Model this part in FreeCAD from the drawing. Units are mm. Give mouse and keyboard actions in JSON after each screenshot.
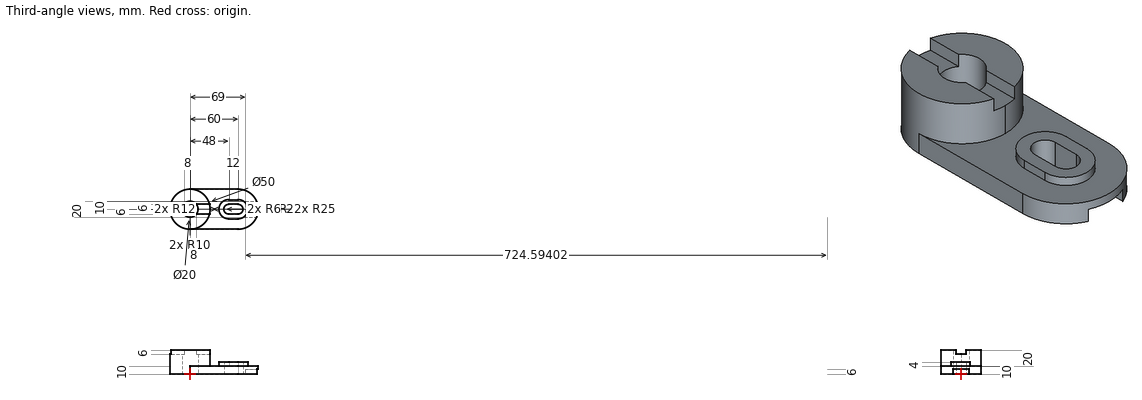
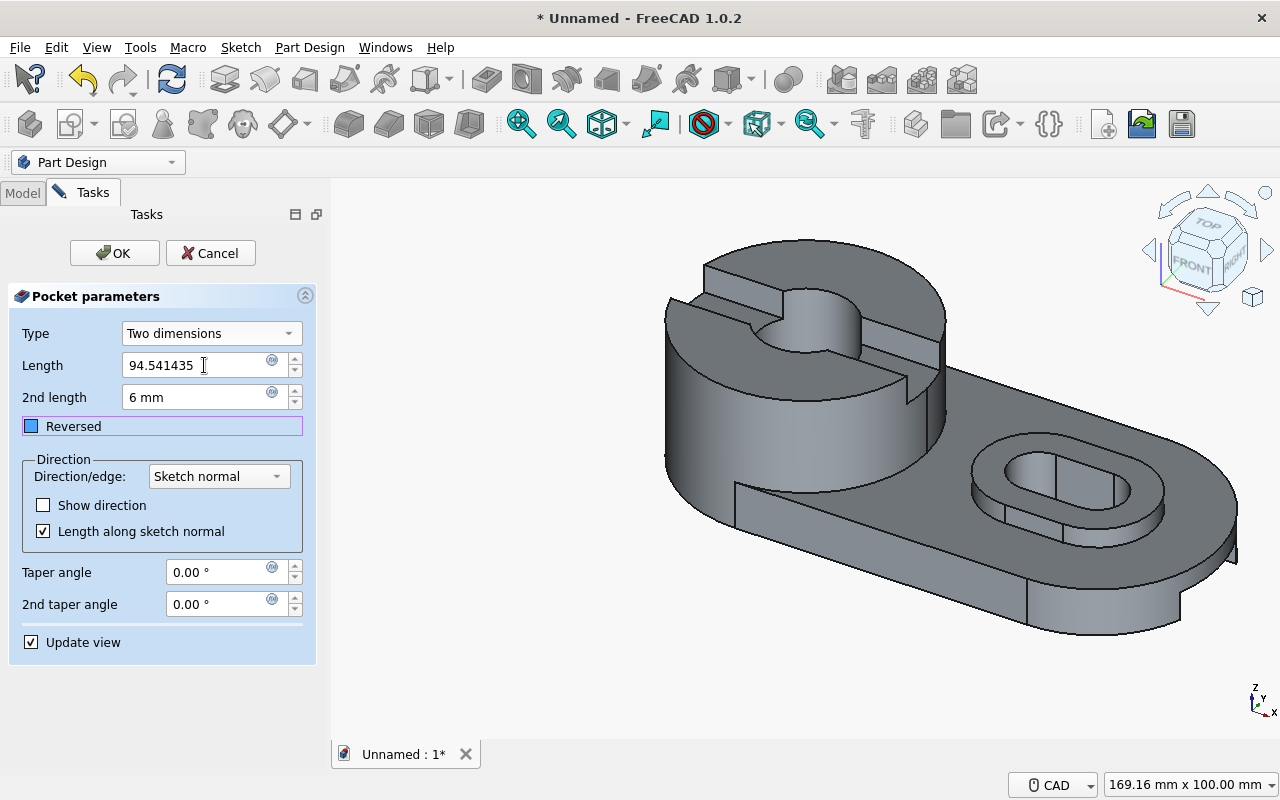
{"action": "left_click", "coordinate": [115, 253]}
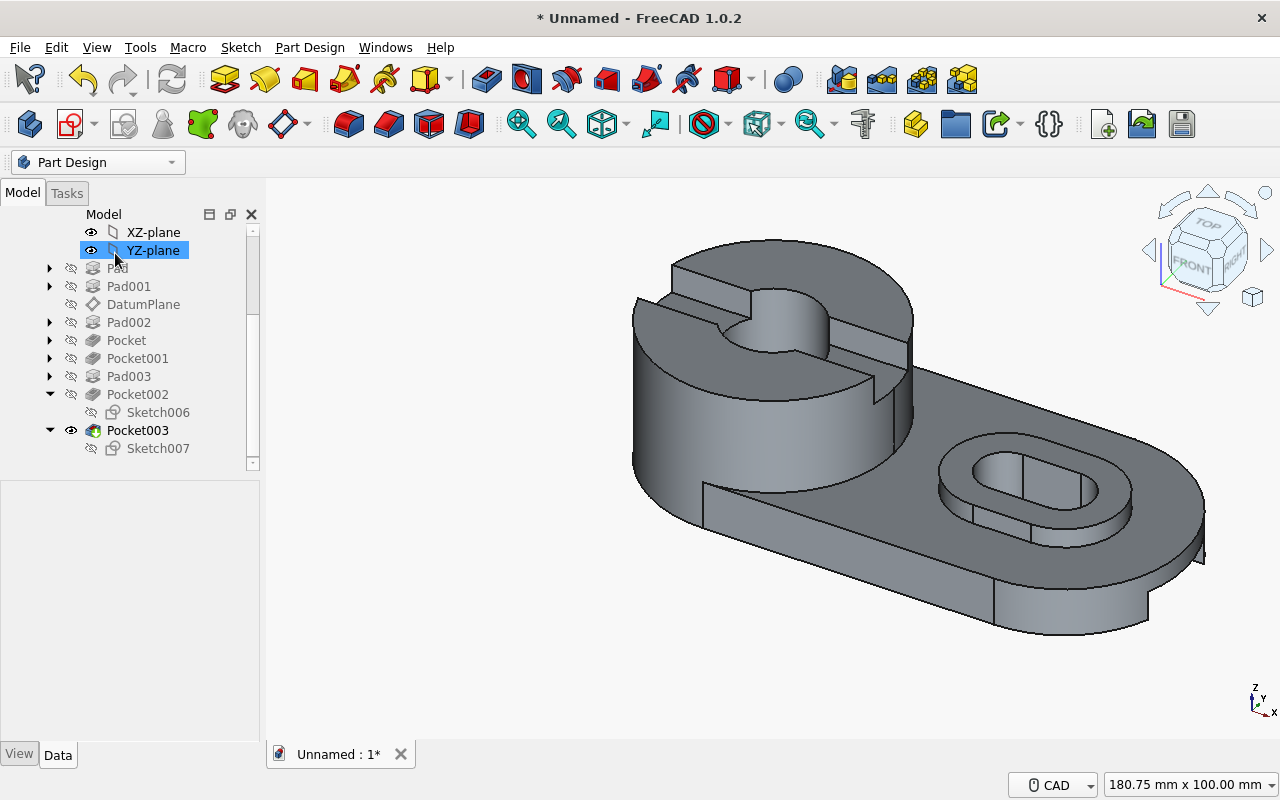
{"action": "key", "text": "0"}